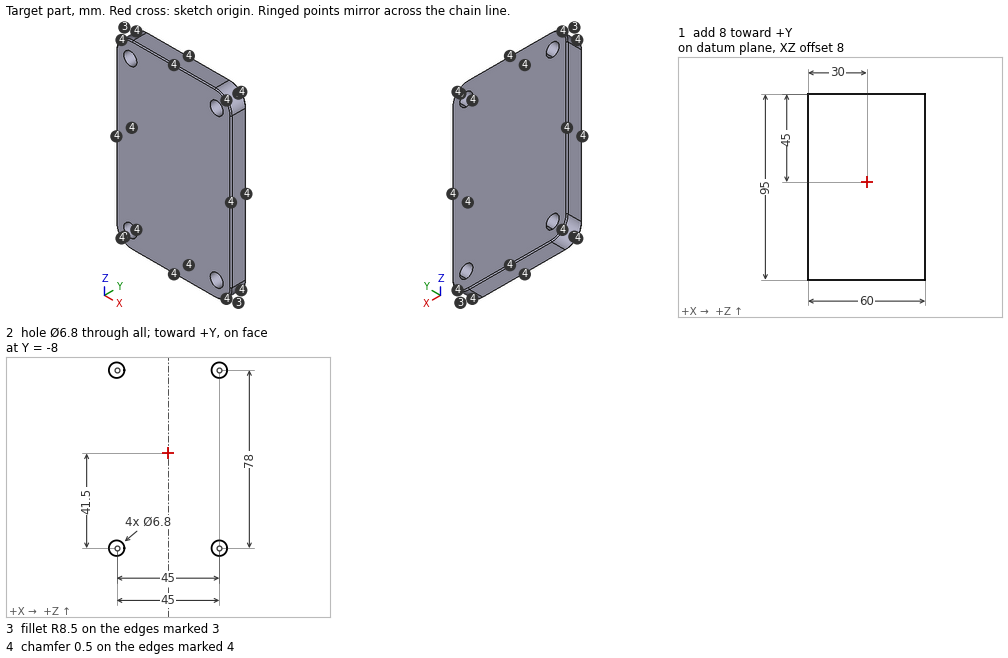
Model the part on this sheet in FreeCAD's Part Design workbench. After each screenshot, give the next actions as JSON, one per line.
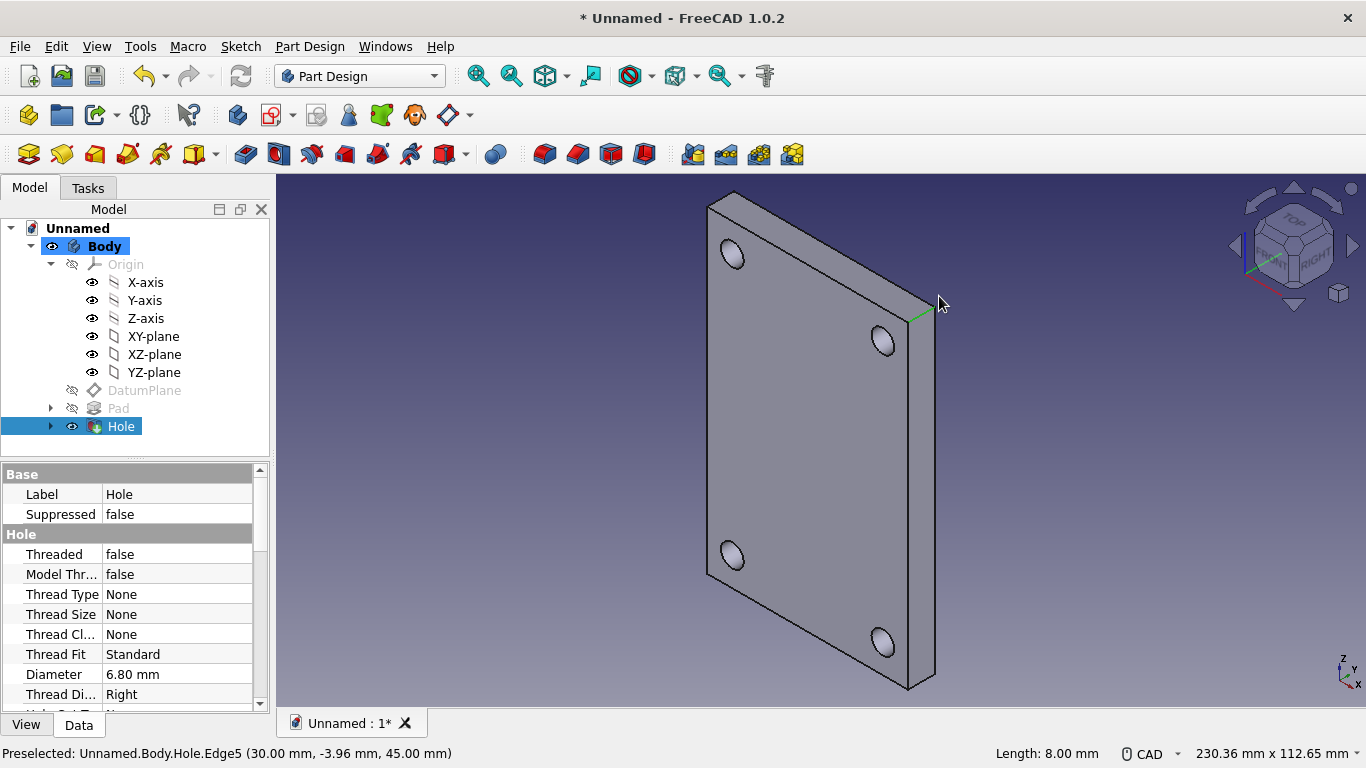
{"action": "key", "text": "2"}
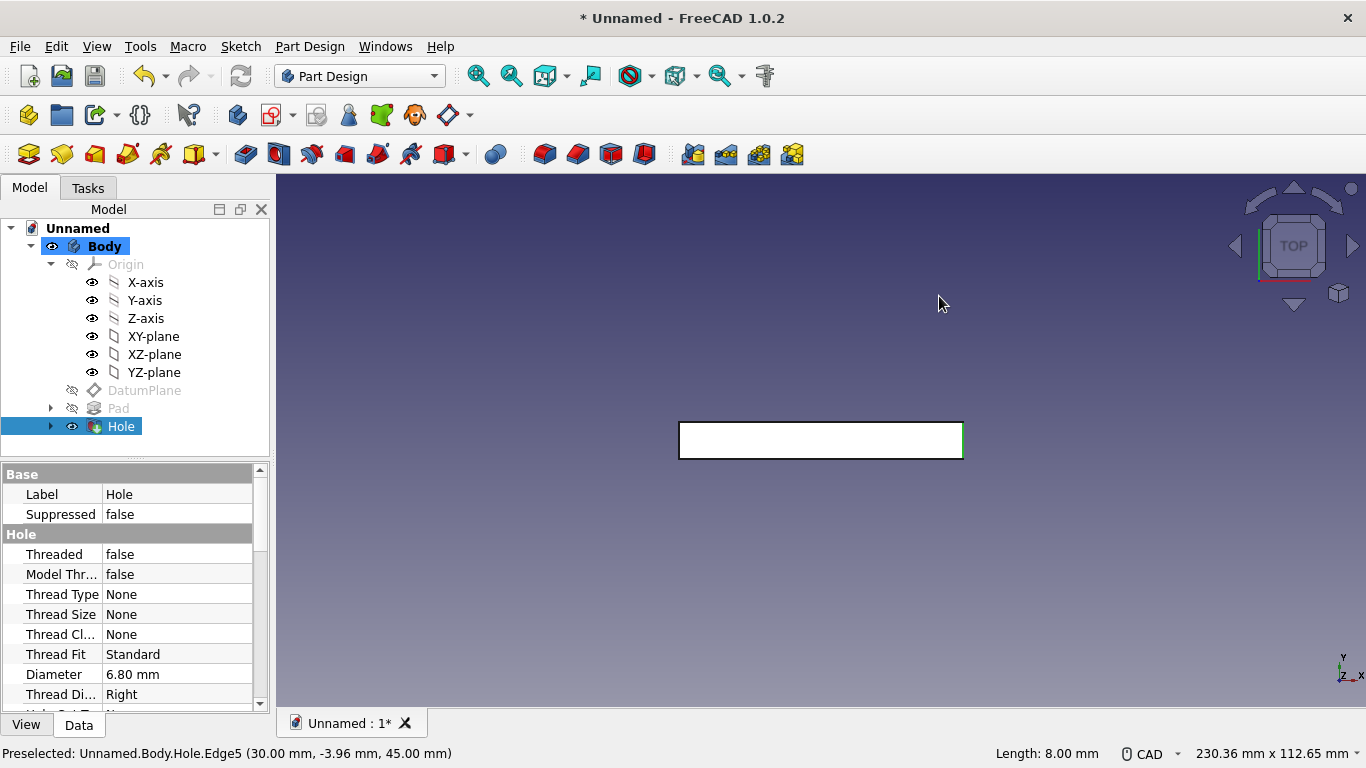
{"action": "left_click", "coordinate": [479, 76]}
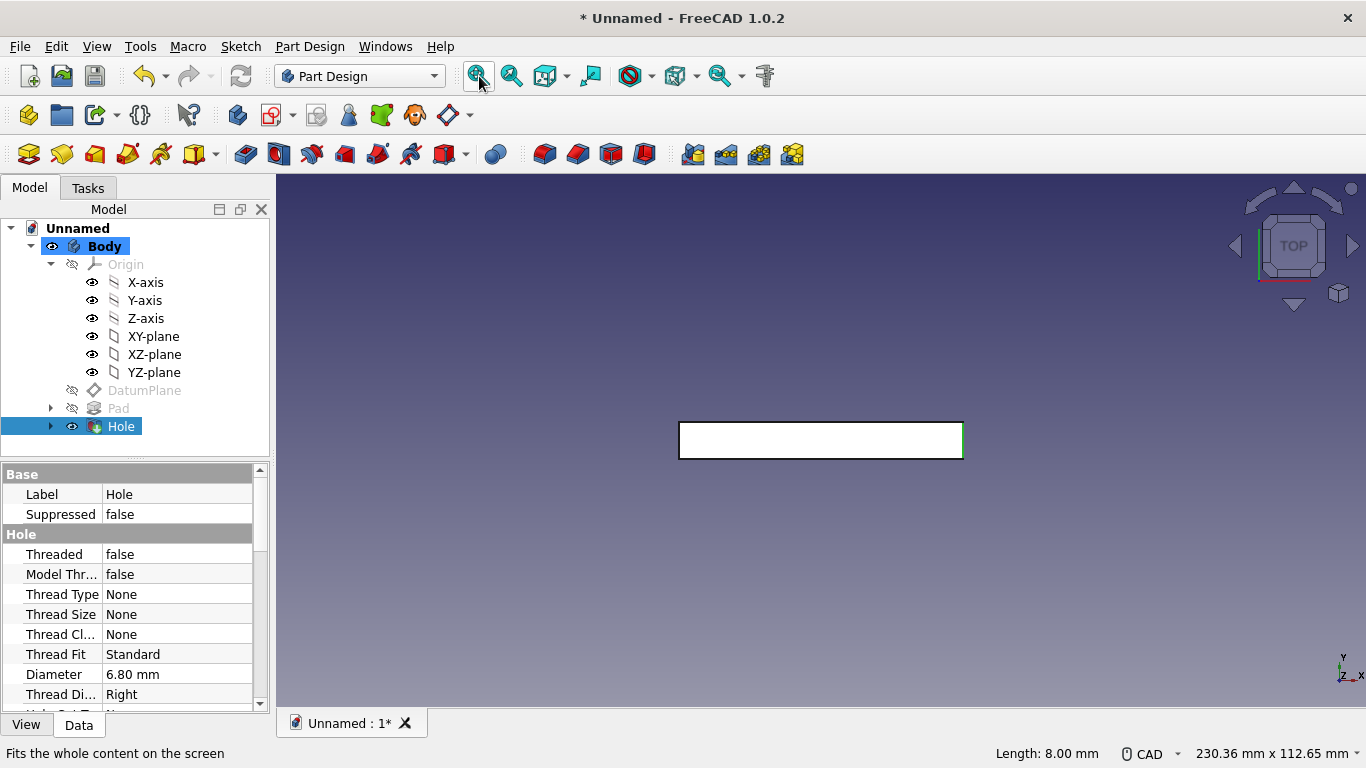
{"action": "left_click", "coordinate": [679, 439], "text": "ctrl"}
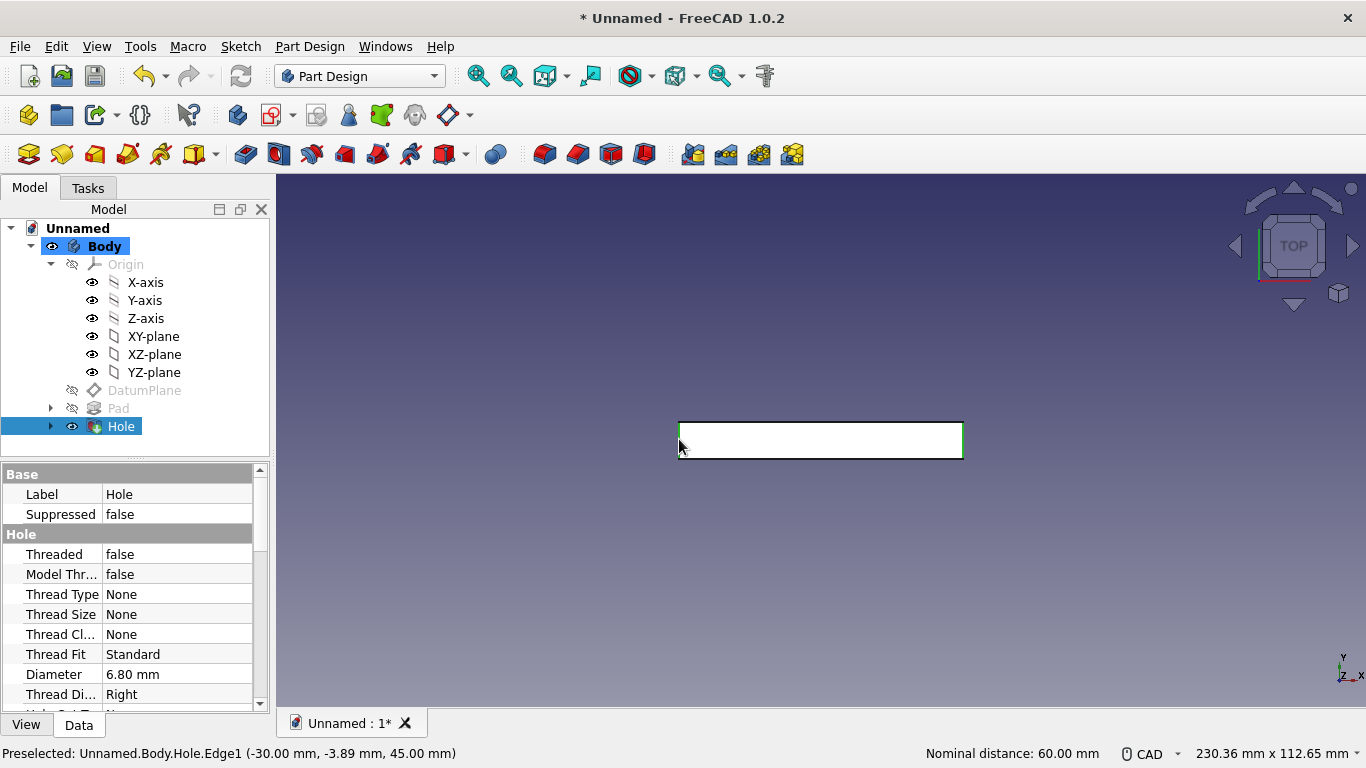
{"action": "key", "text": "1"}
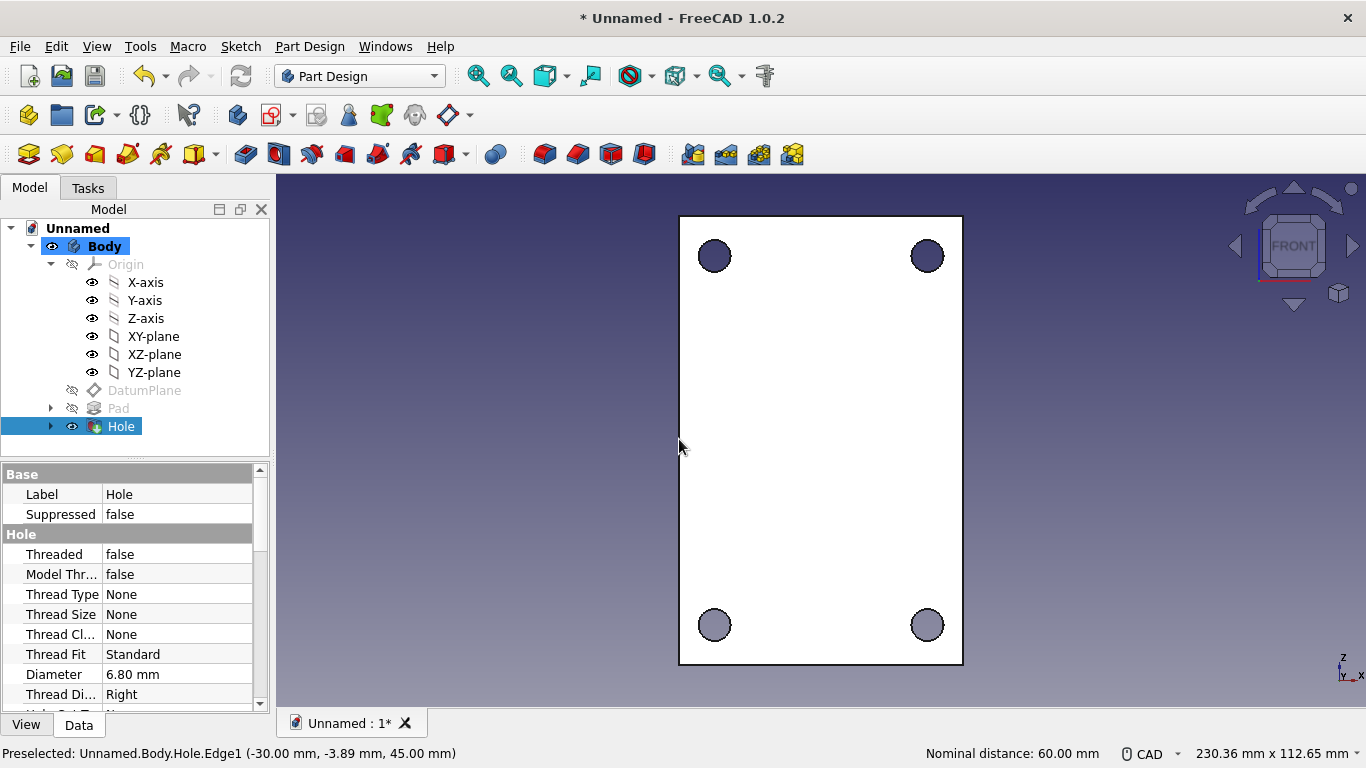
{"action": "key", "text": "3"}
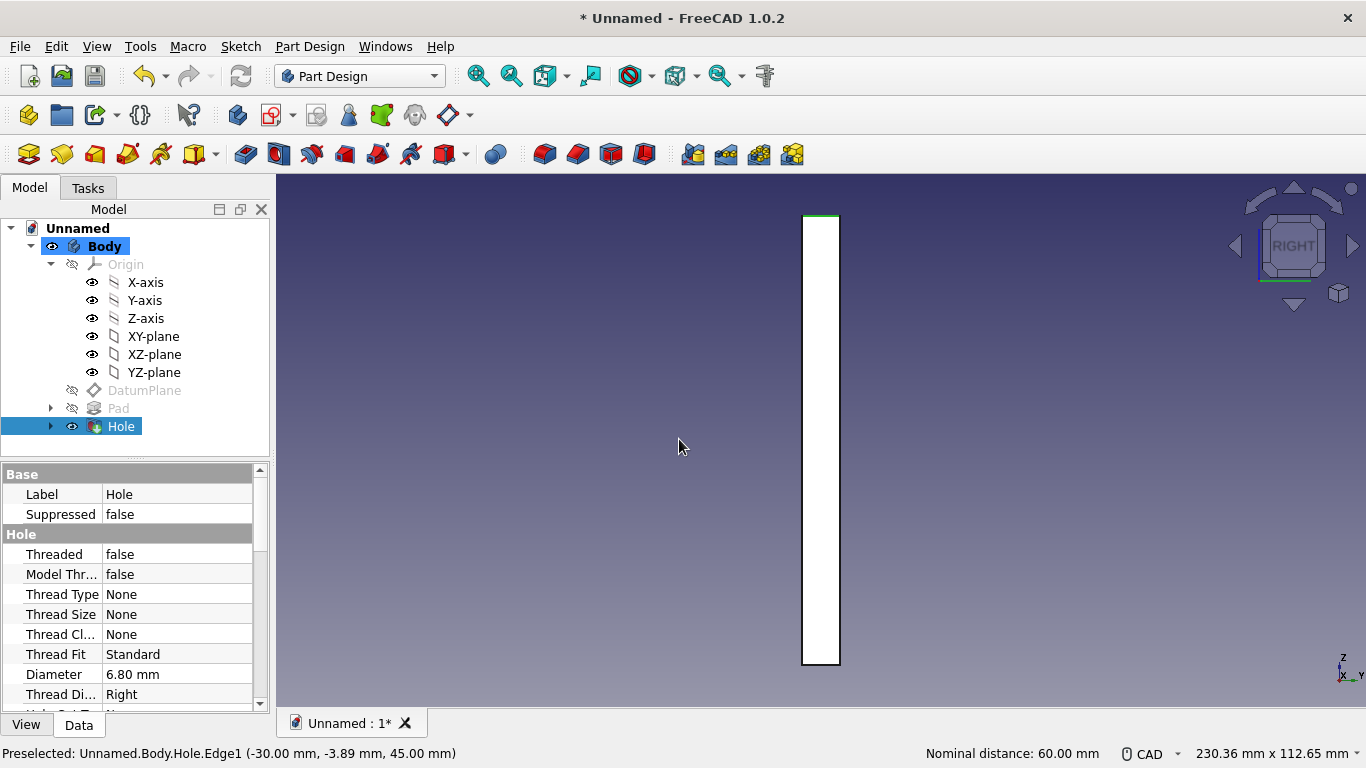
{"action": "left_click", "coordinate": [821, 664], "text": "ctrl"}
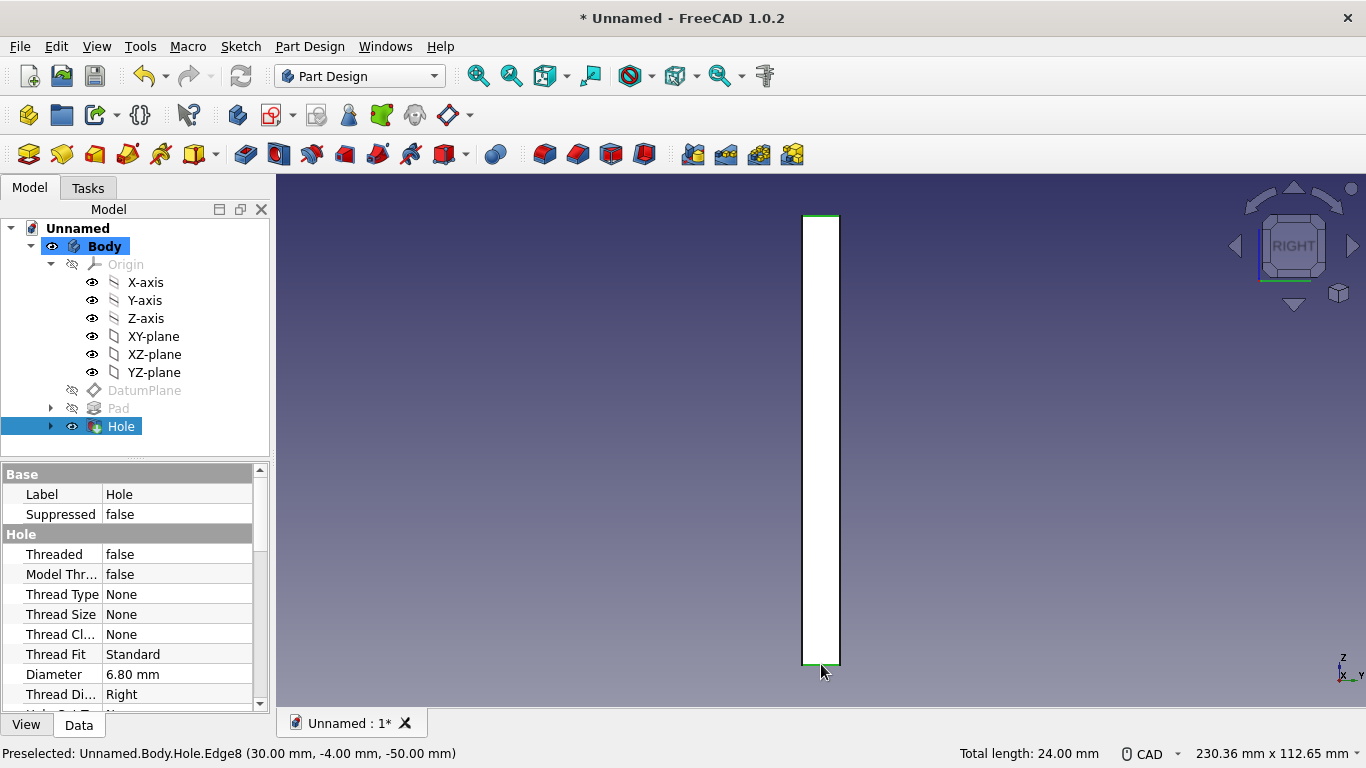
{"action": "key", "text": "5"}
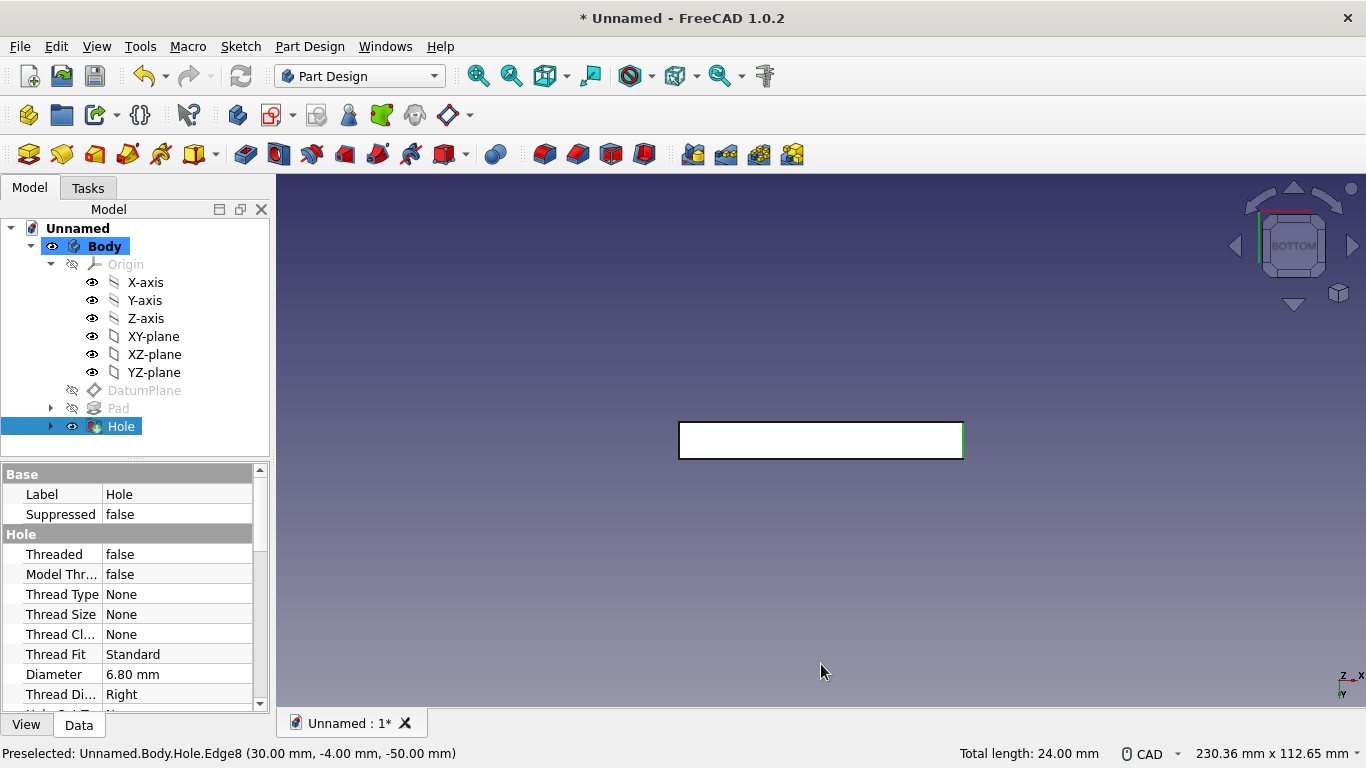
{"action": "left_click", "coordinate": [479, 76]}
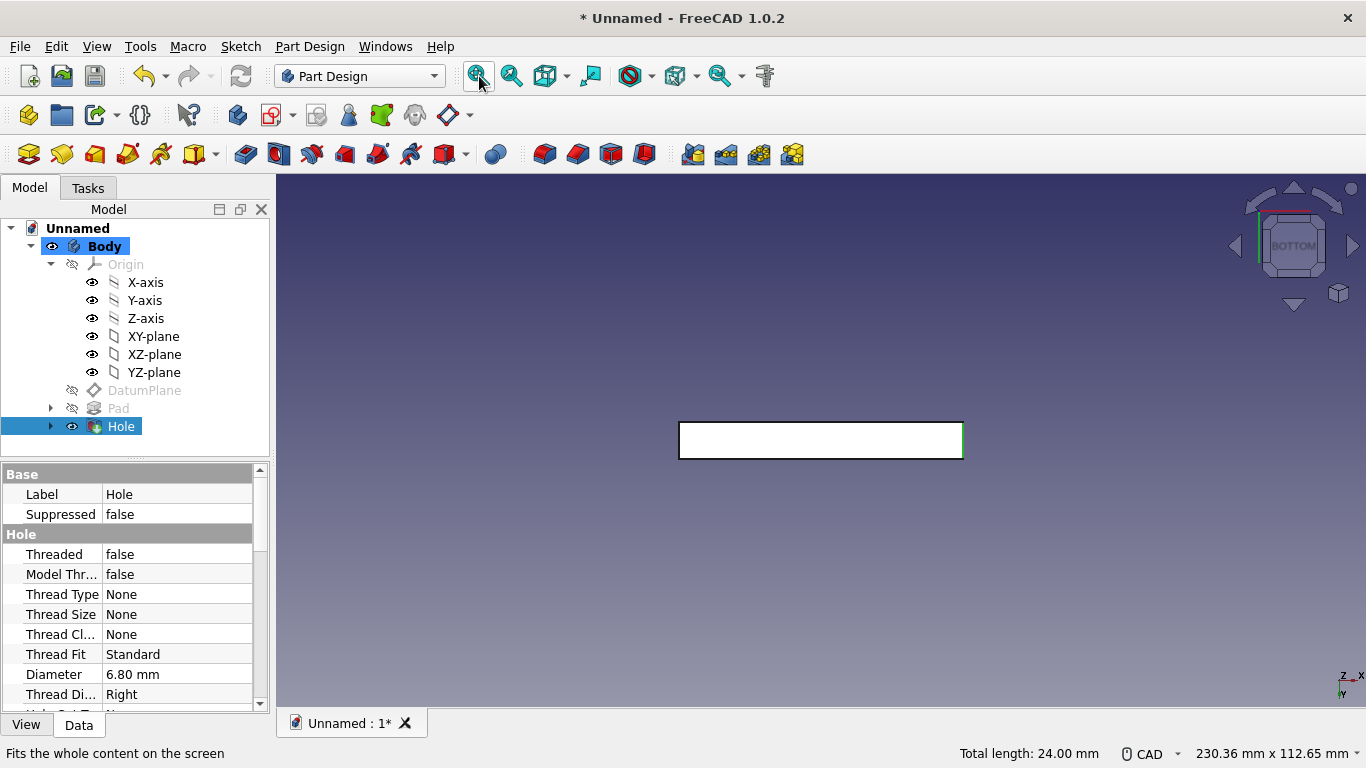
{"action": "left_click", "coordinate": [679, 439], "text": "ctrl"}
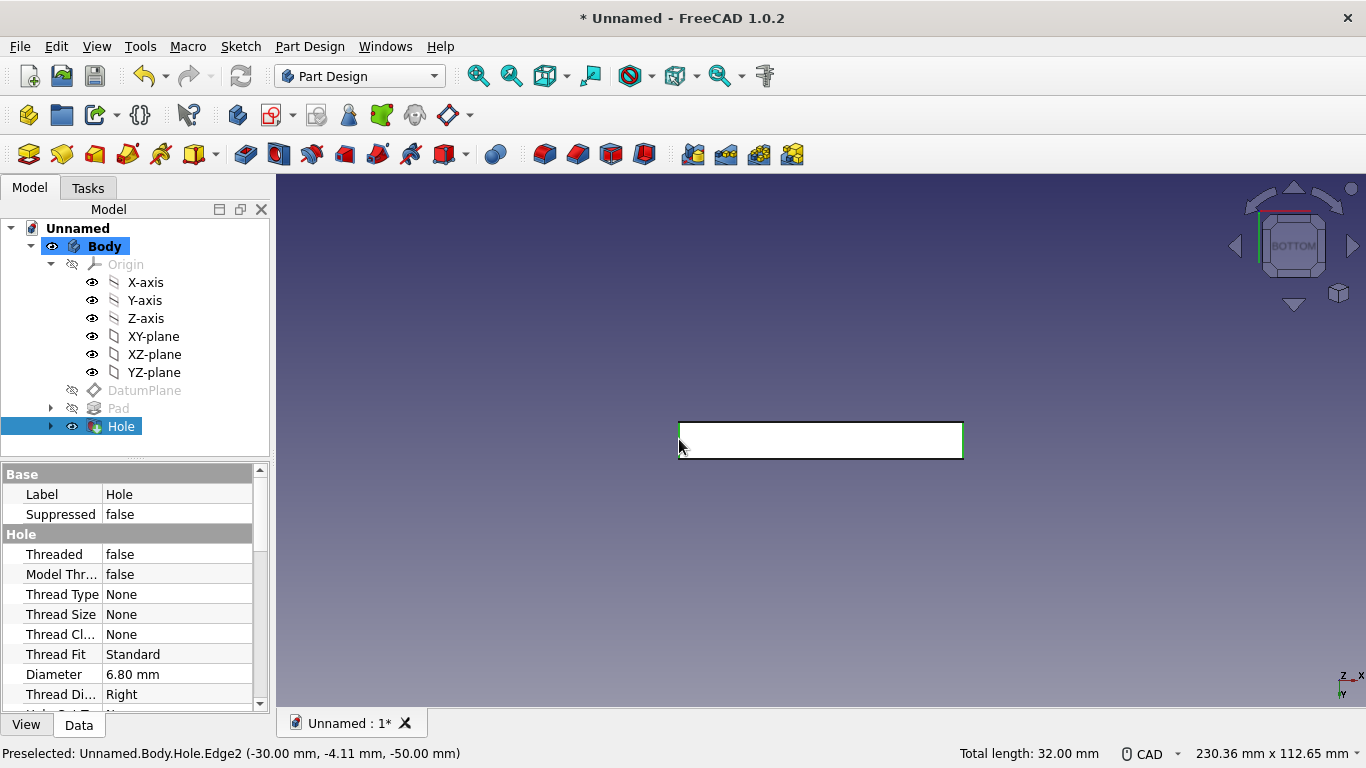
{"action": "left_click", "coordinate": [545, 154]}